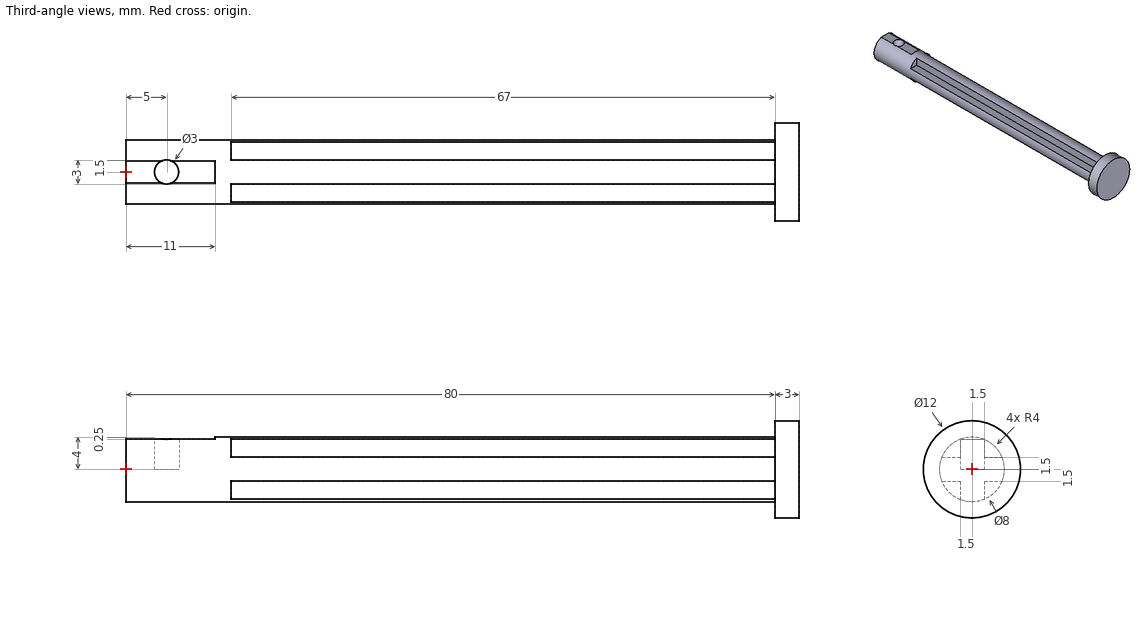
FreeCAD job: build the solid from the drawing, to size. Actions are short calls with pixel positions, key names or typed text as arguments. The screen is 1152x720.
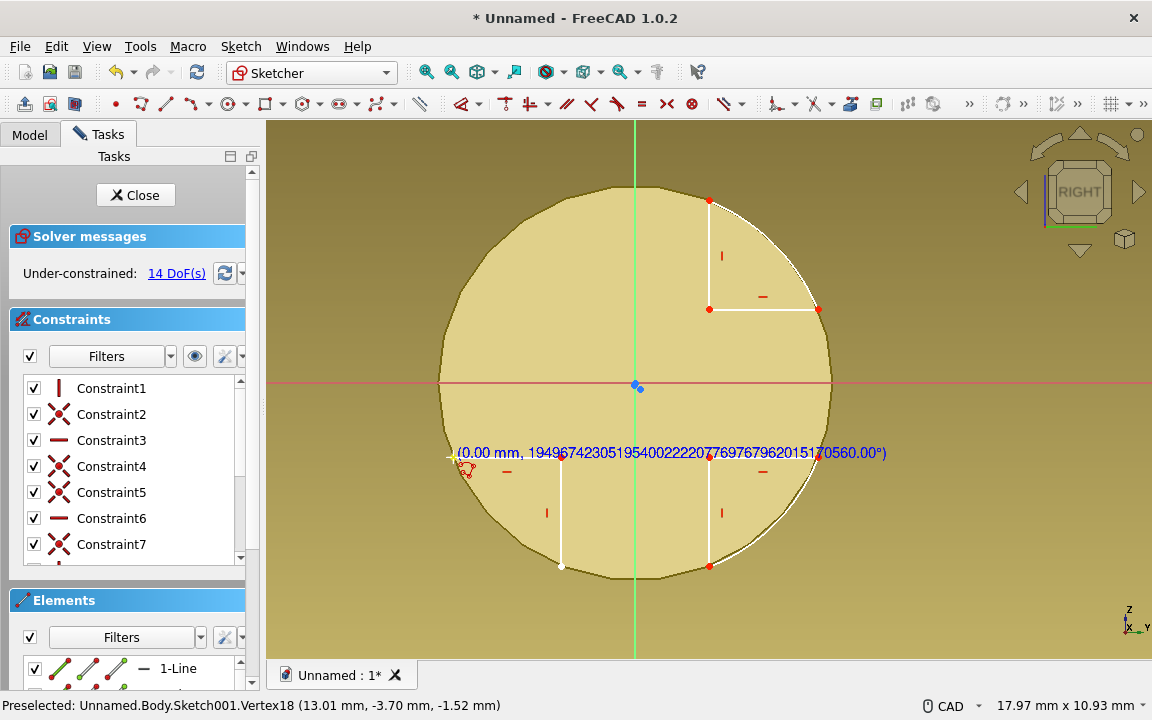
key(g)
key(3)
key(a)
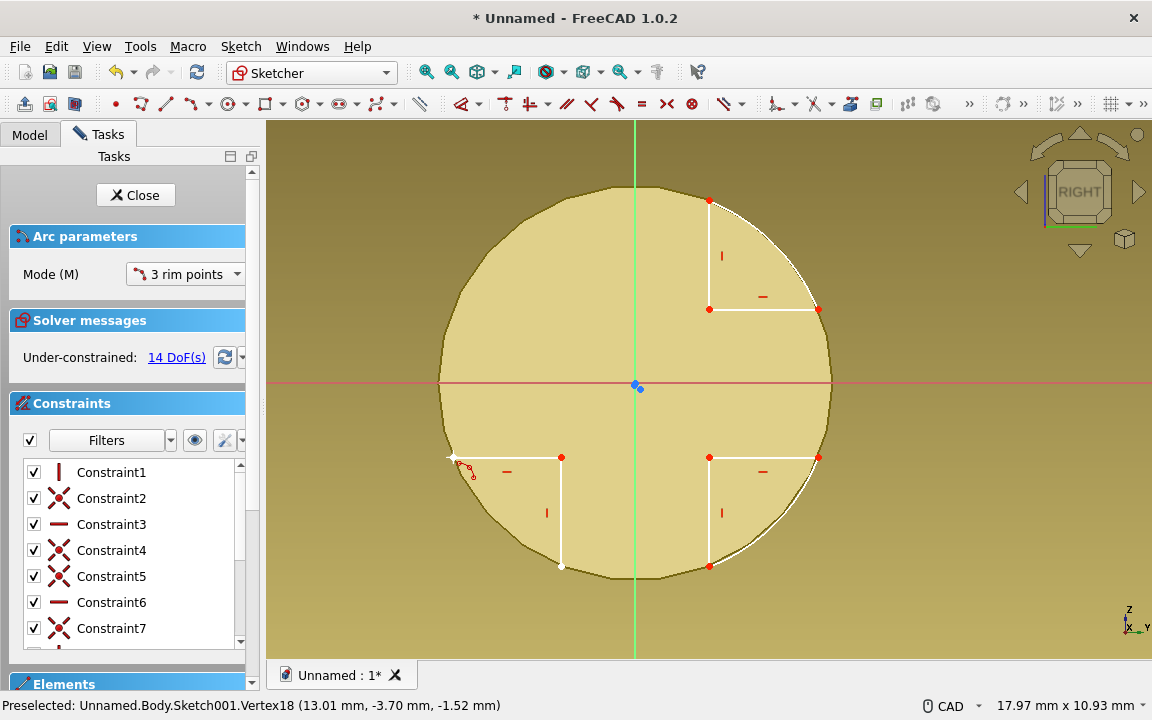
click(453, 458)
click(561, 567)
click(496, 523)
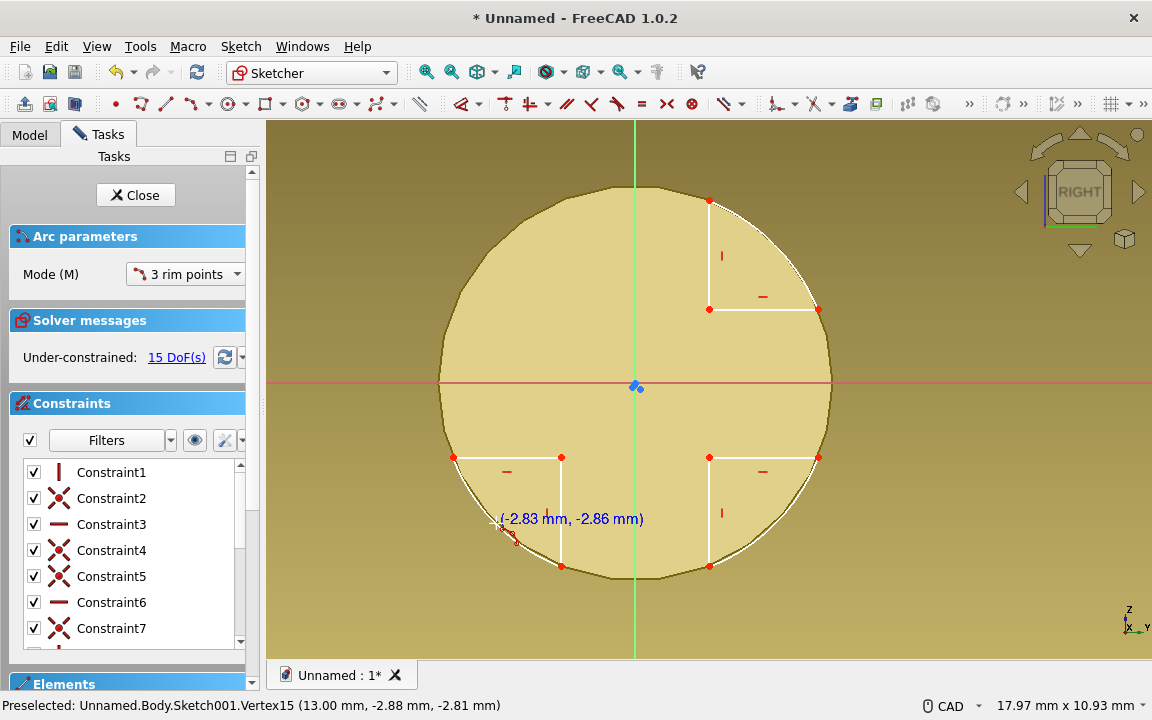
key(g)
key(m)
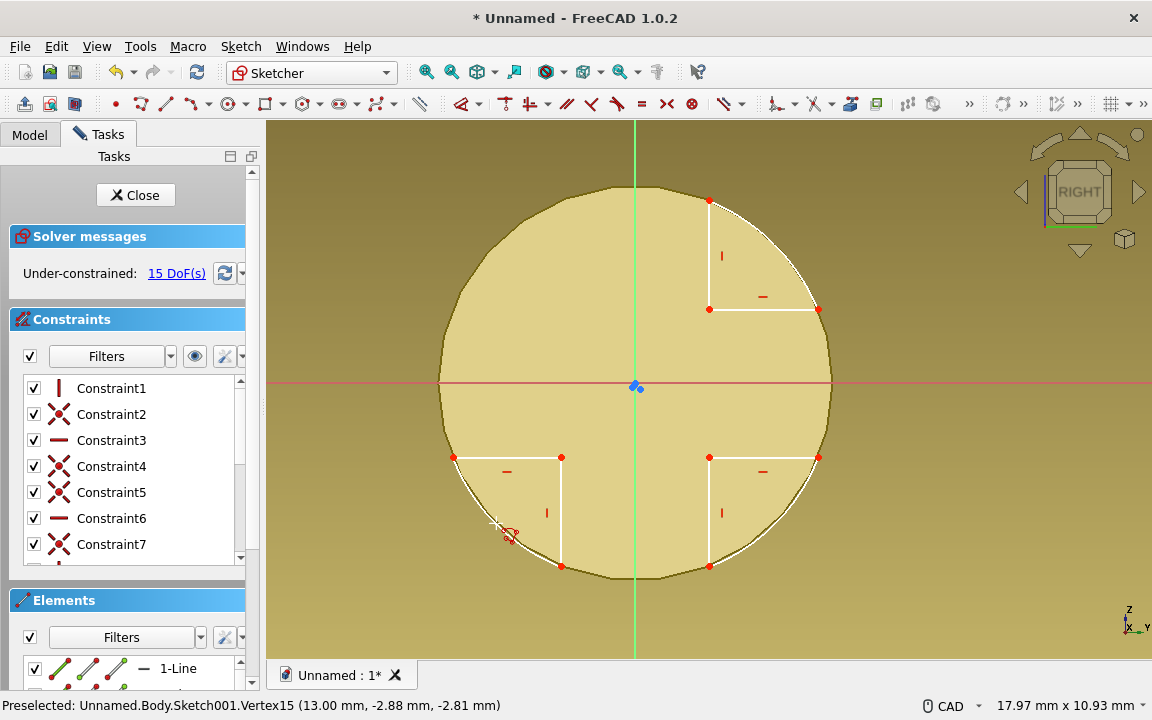
click(453, 309)
click(561, 309)
click(561, 200)
right_click(561, 200)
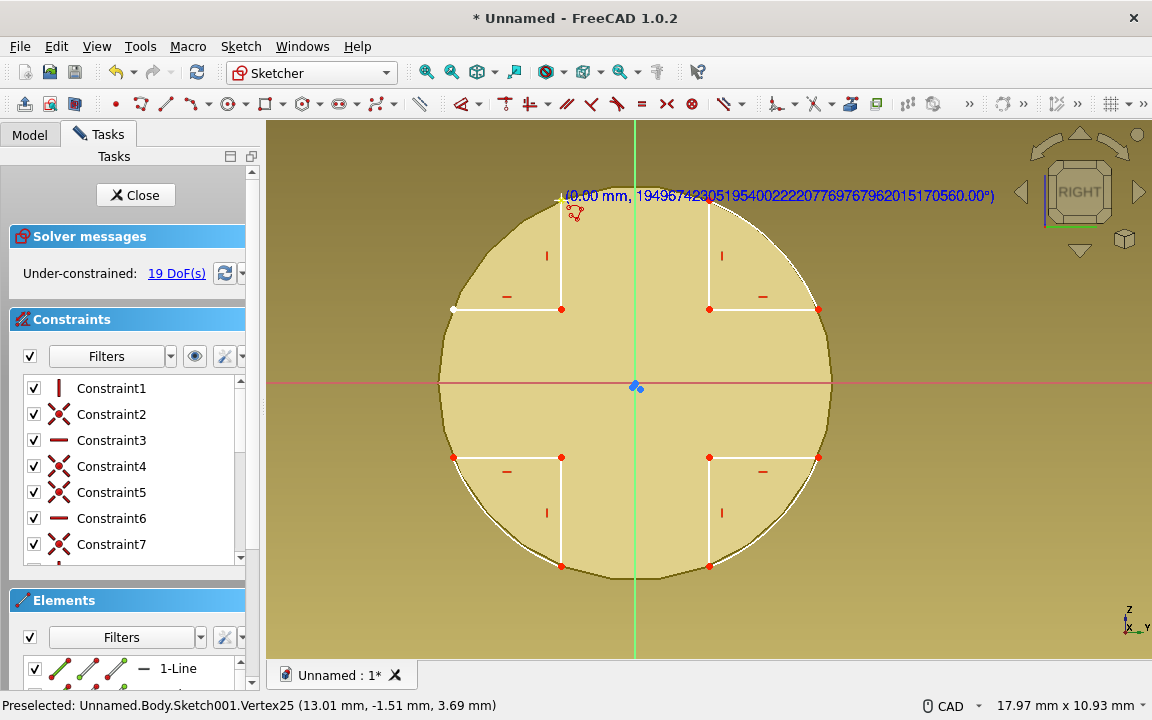
click(190, 104)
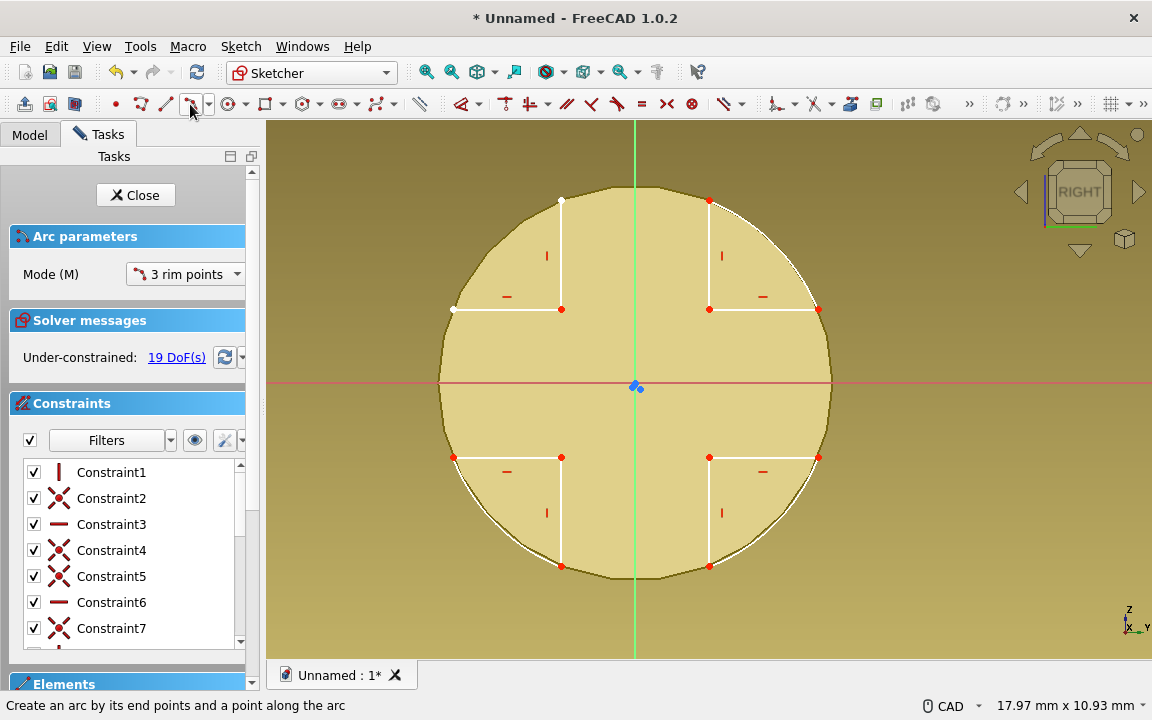
click(561, 201)
click(453, 310)
click(496, 244)
key(Escape)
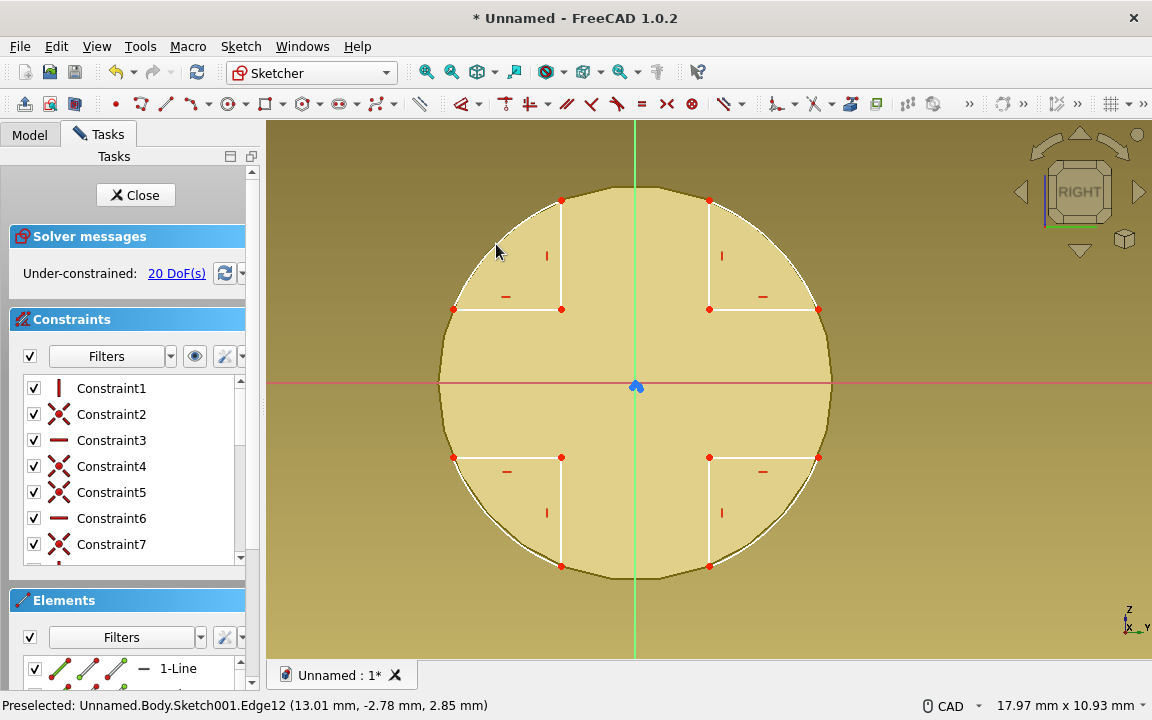
click(795, 269)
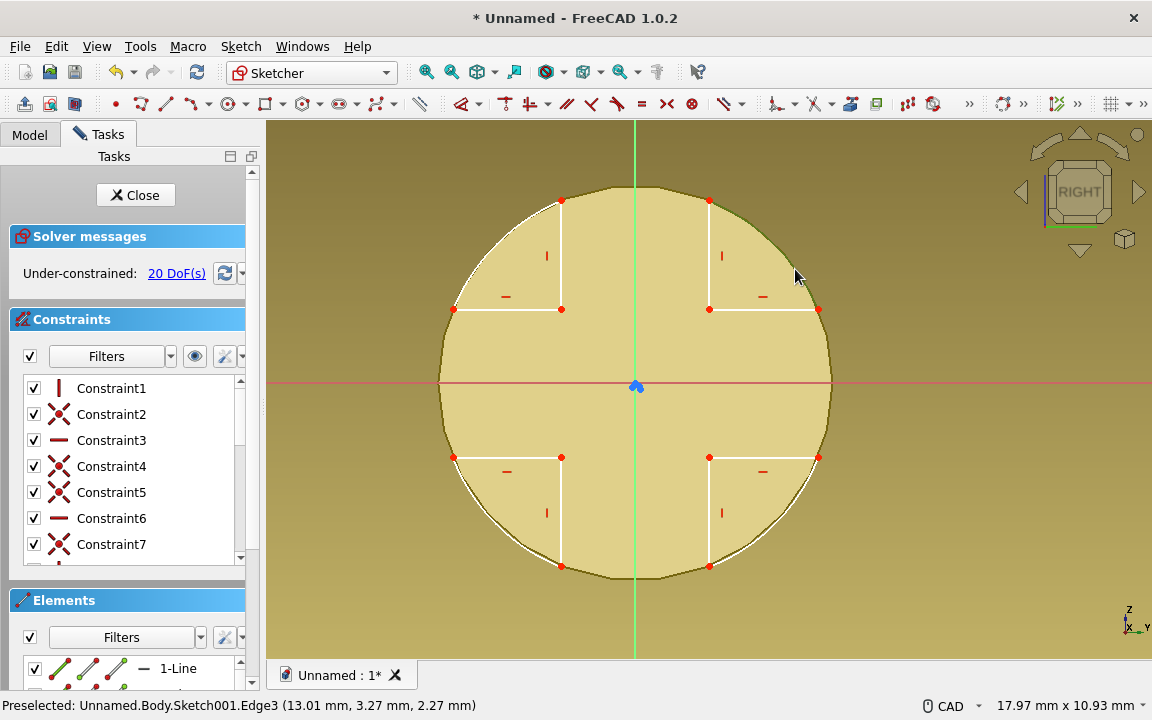
click(751, 544)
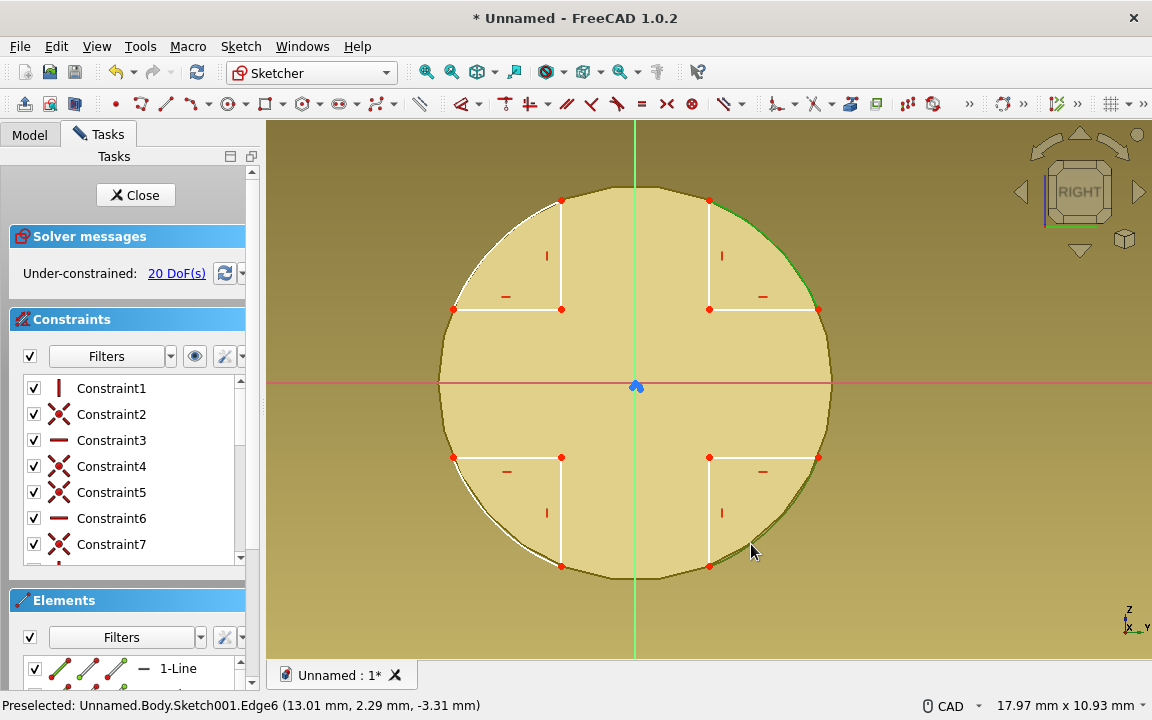
key(c)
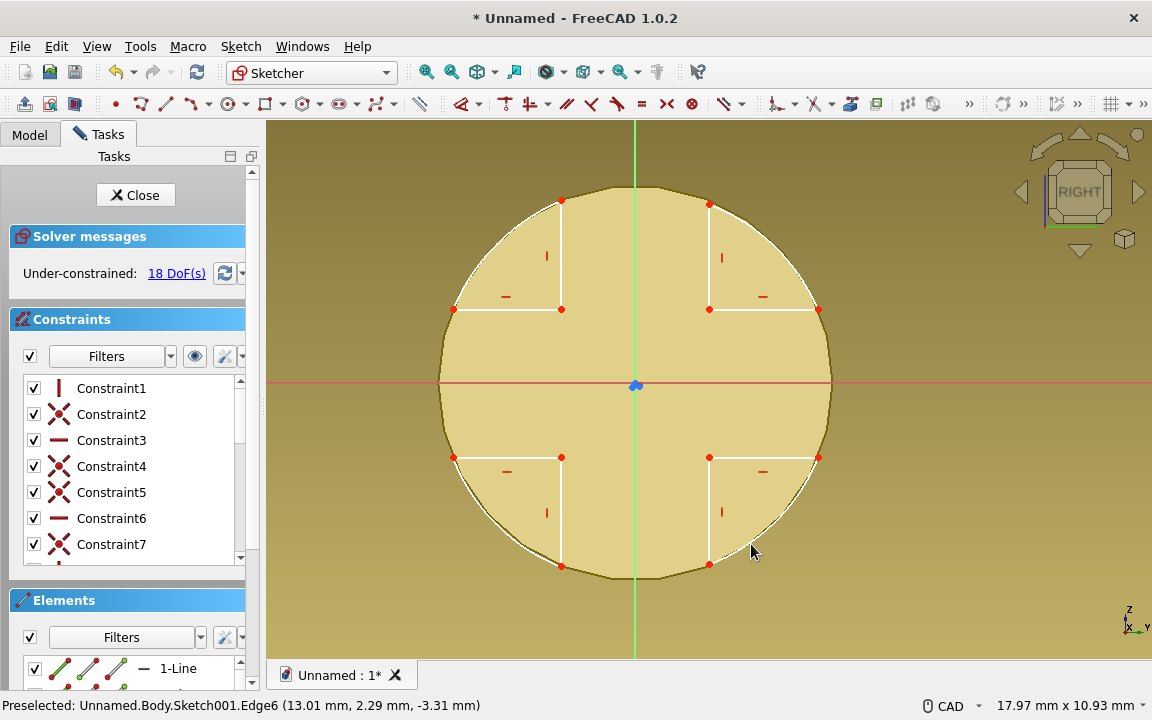
click(795, 270)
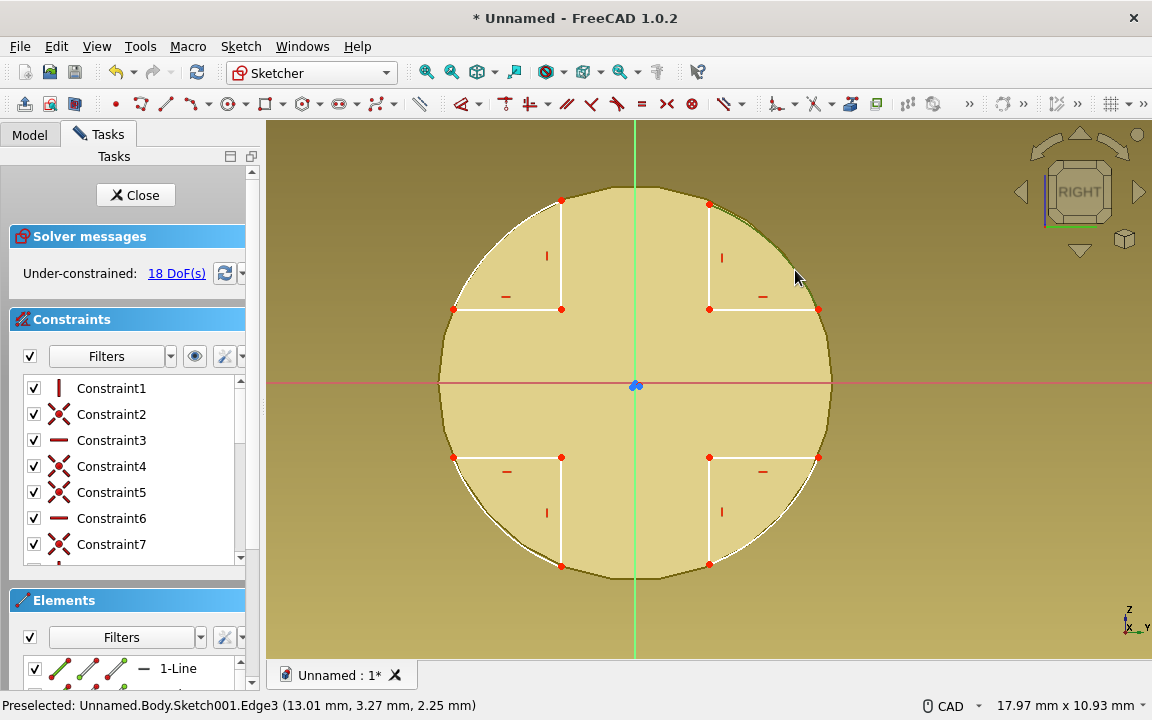
click(475, 500)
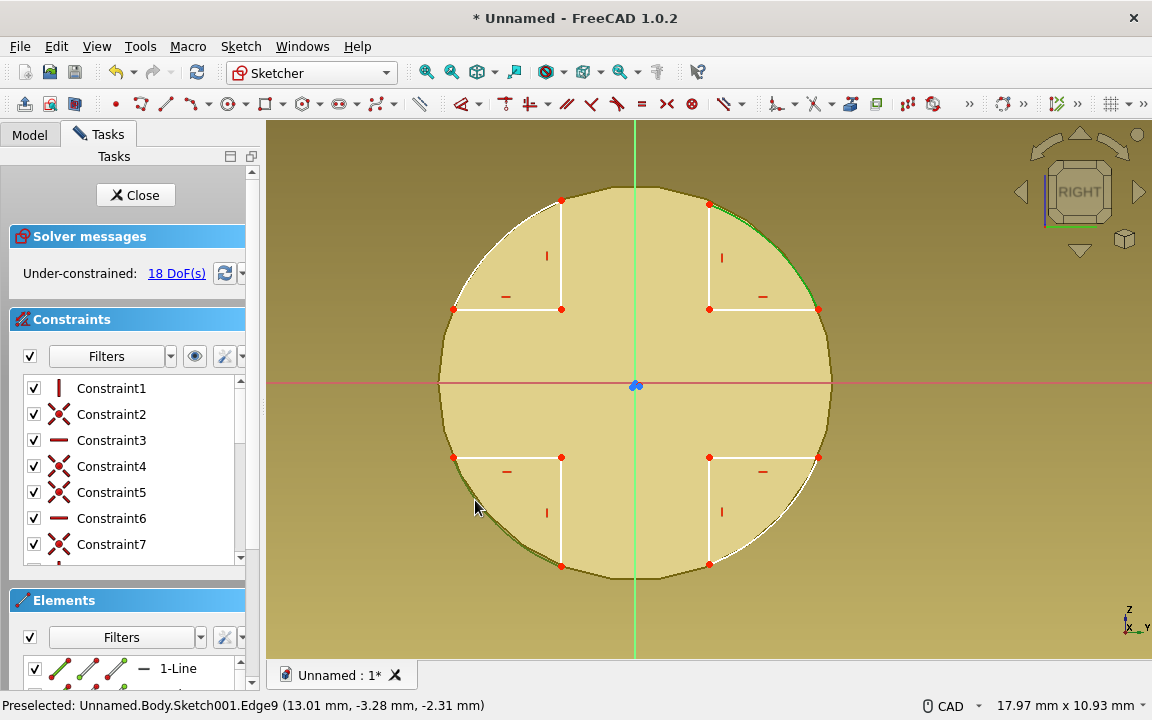
key(c)